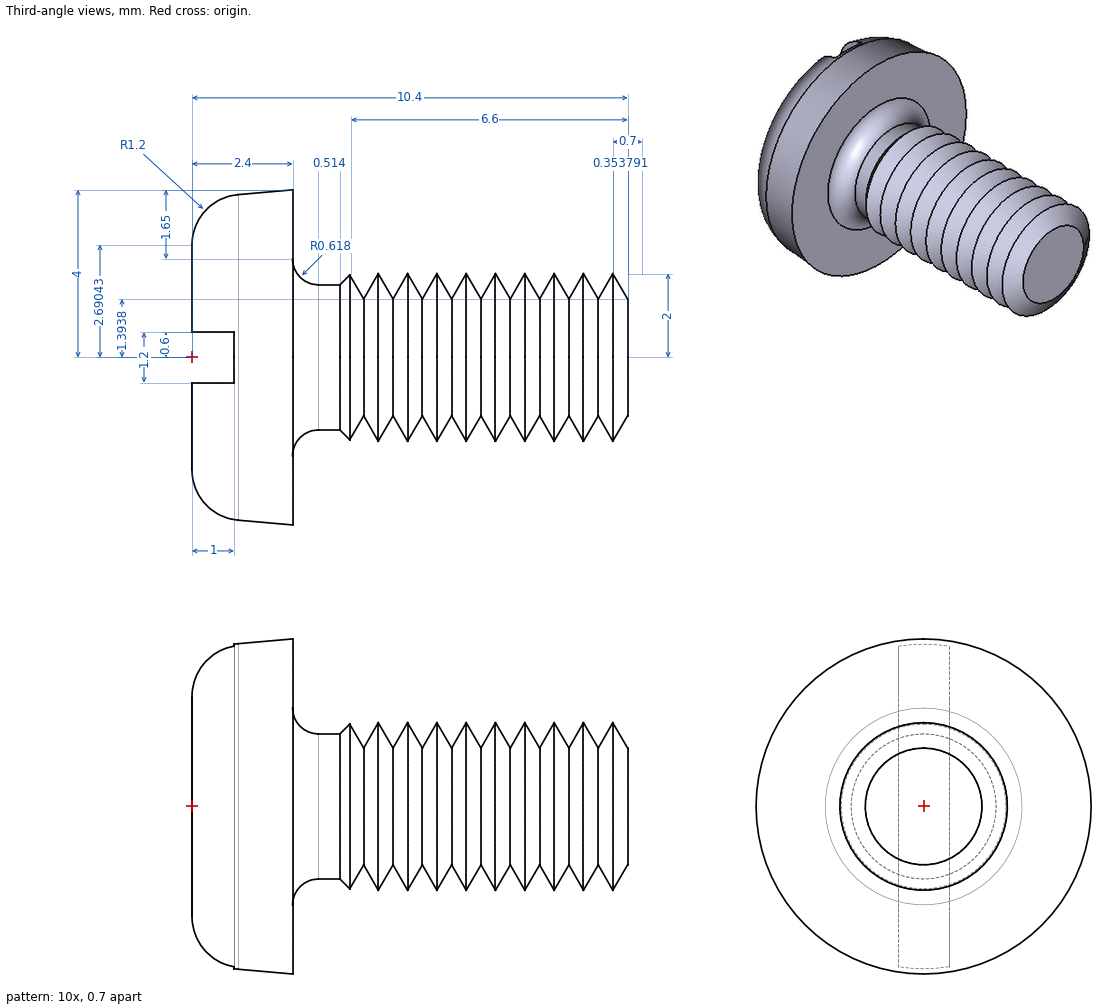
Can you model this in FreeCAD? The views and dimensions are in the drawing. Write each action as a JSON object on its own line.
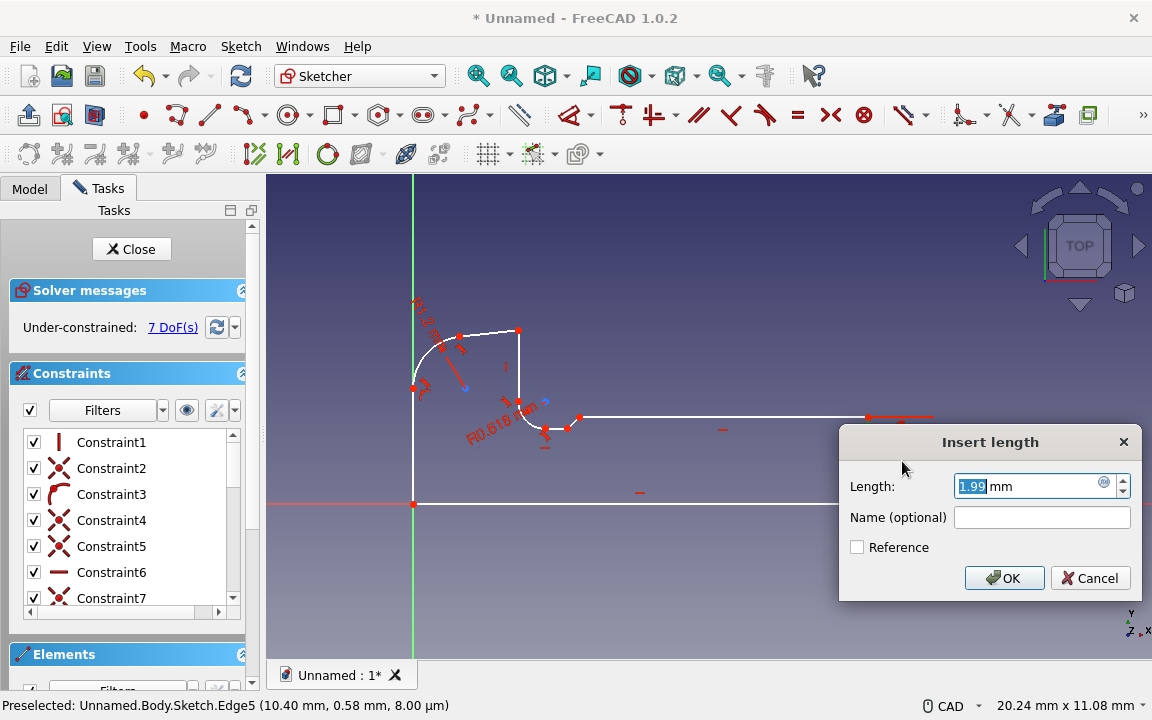
{"action": "type", "text": "2"}
{"action": "key", "text": "Return"}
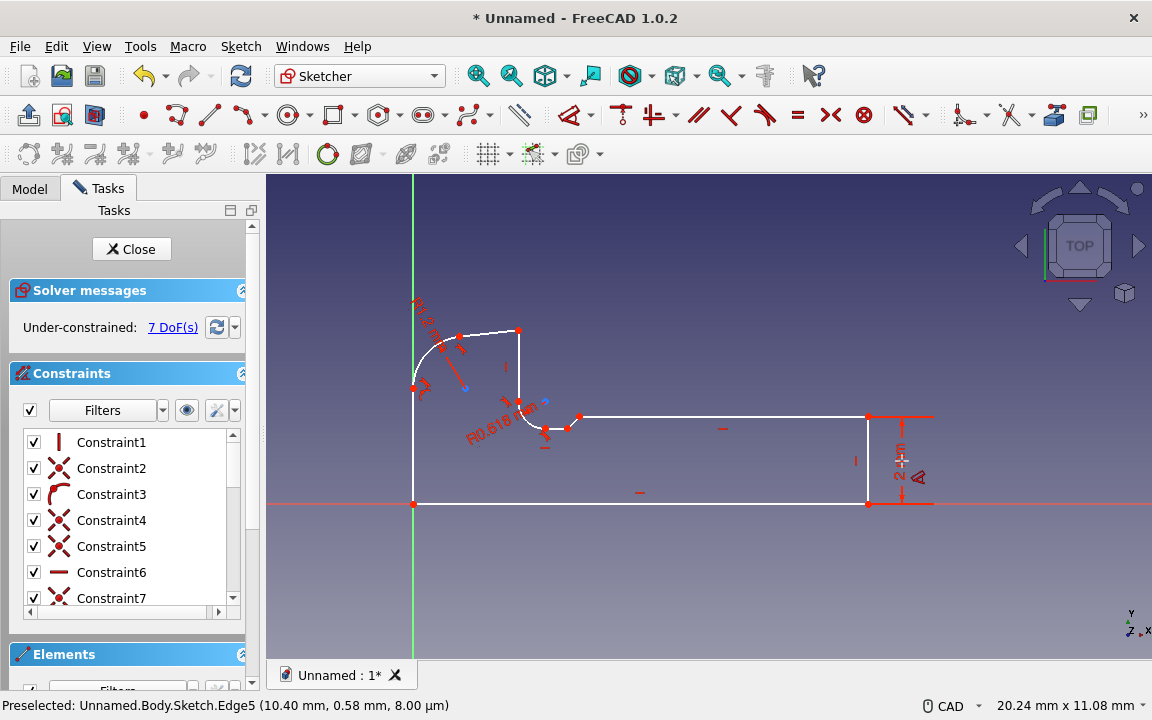
{"action": "left_click", "coordinate": [519, 330]}
{"action": "left_click", "coordinate": [379, 417]}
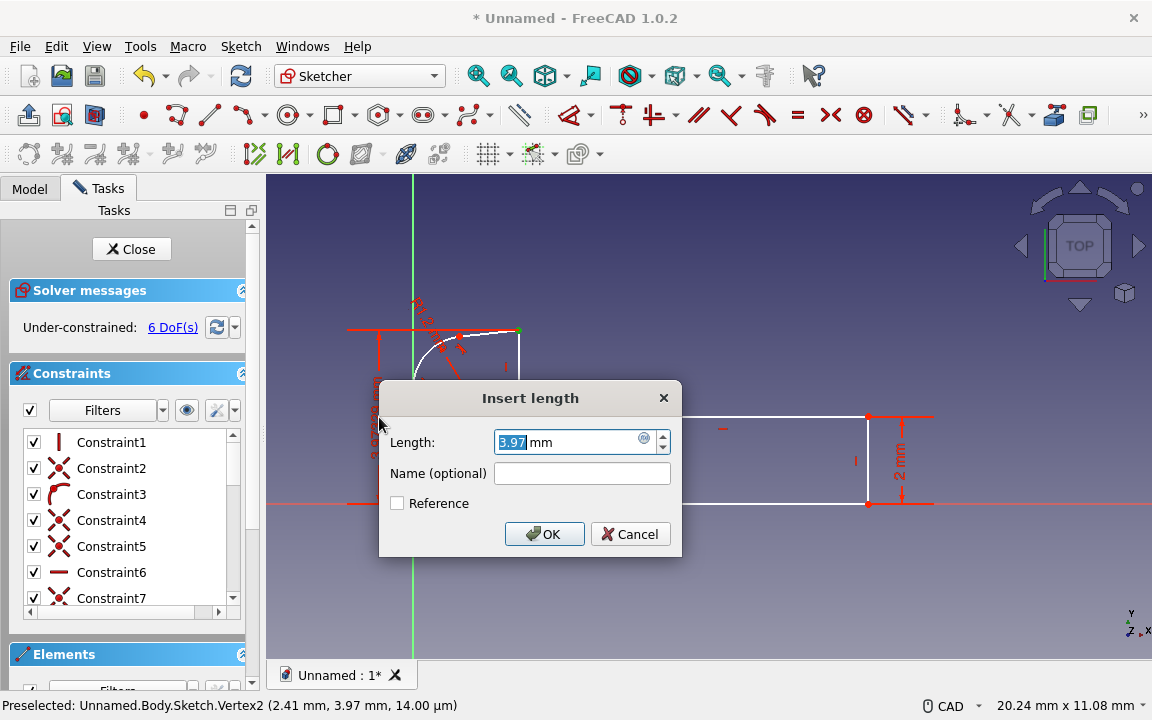
{"action": "type", "text": "4"}
{"action": "key", "text": "Return"}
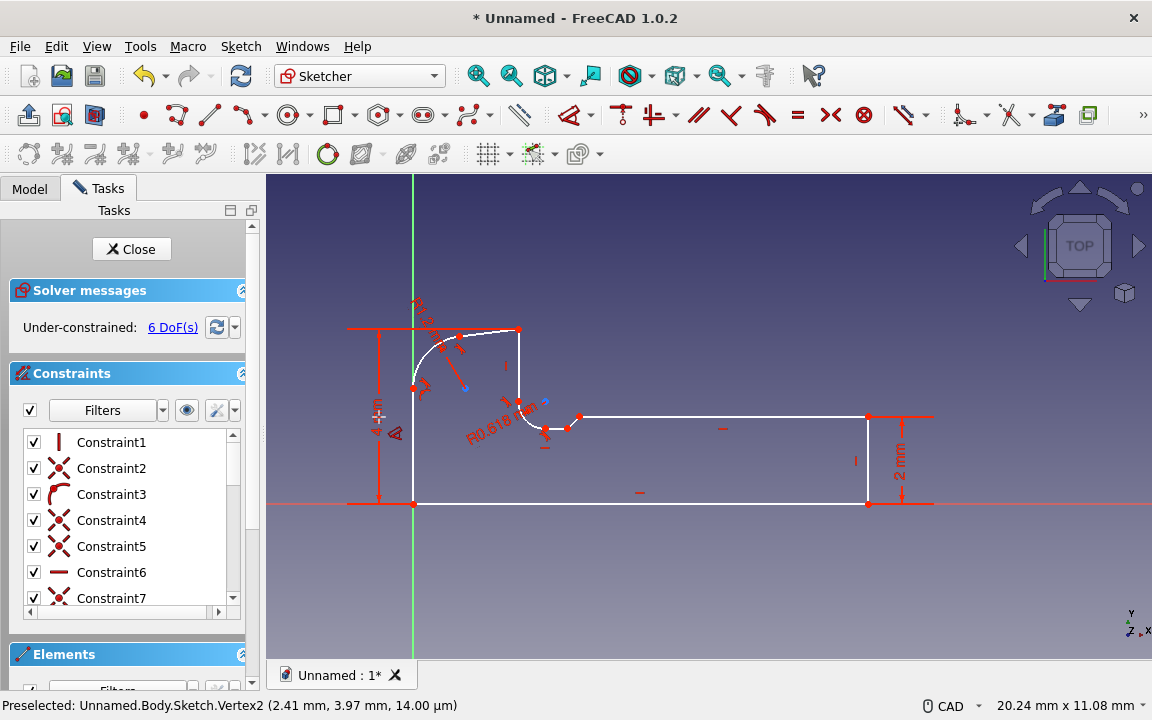
{"action": "left_click", "coordinate": [782, 417]}
{"action": "left_click", "coordinate": [724, 451]}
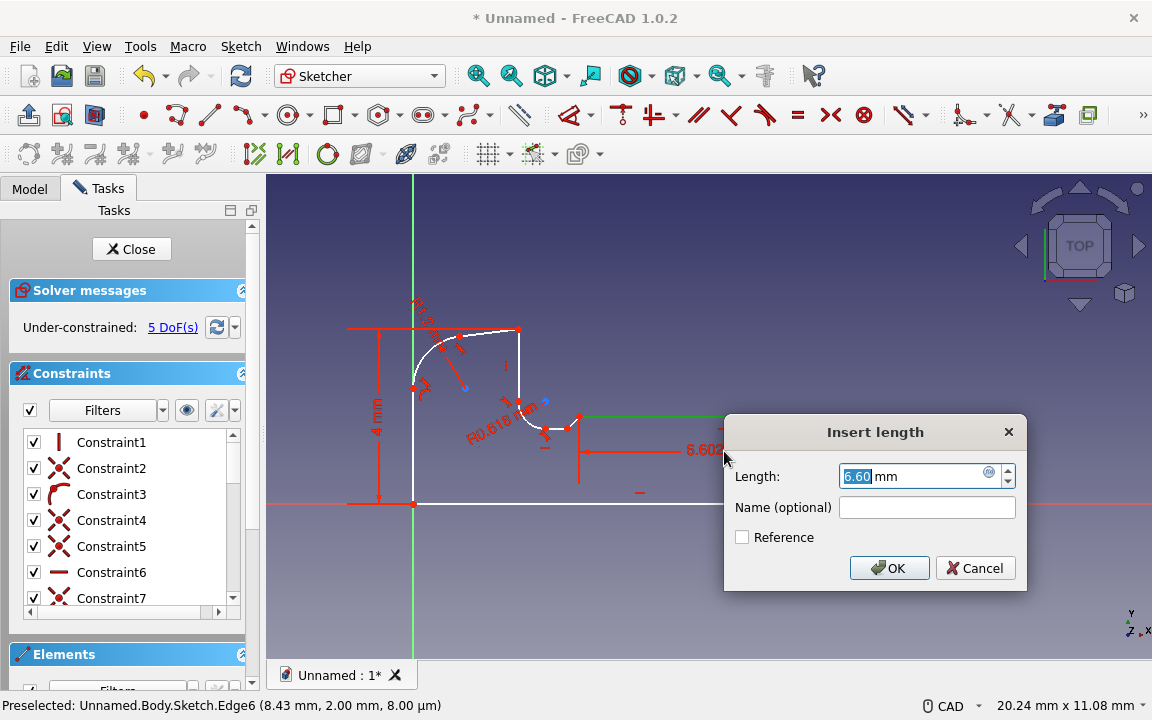
{"action": "type", "text": "6.6"}
{"action": "key", "text": "Return"}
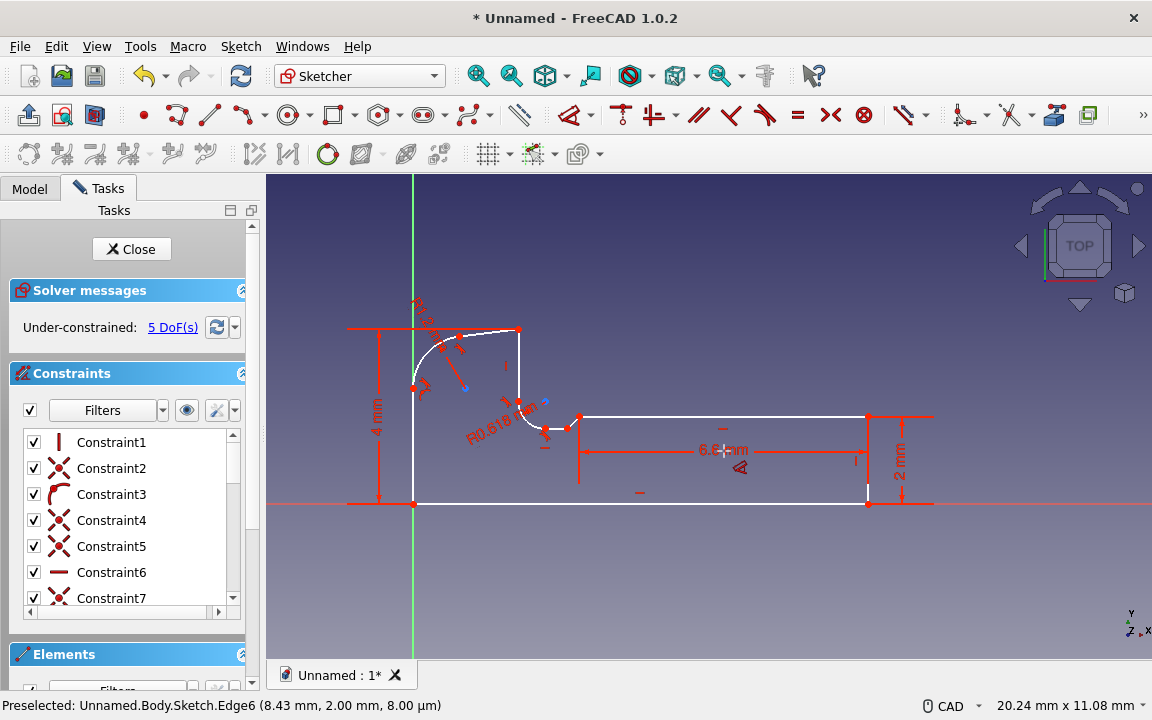
{"action": "left_click", "coordinate": [519, 380]}
{"action": "left_click", "coordinate": [485, 366]}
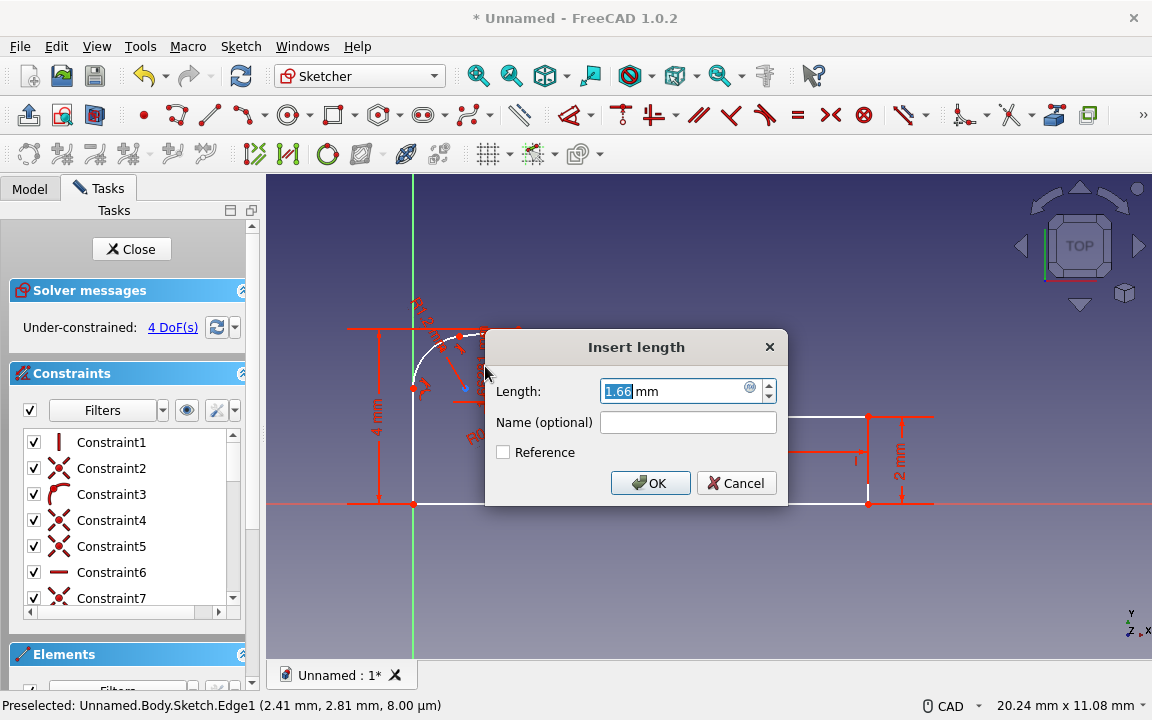
{"action": "type", "text": "1.65"}
{"action": "key", "text": "Return"}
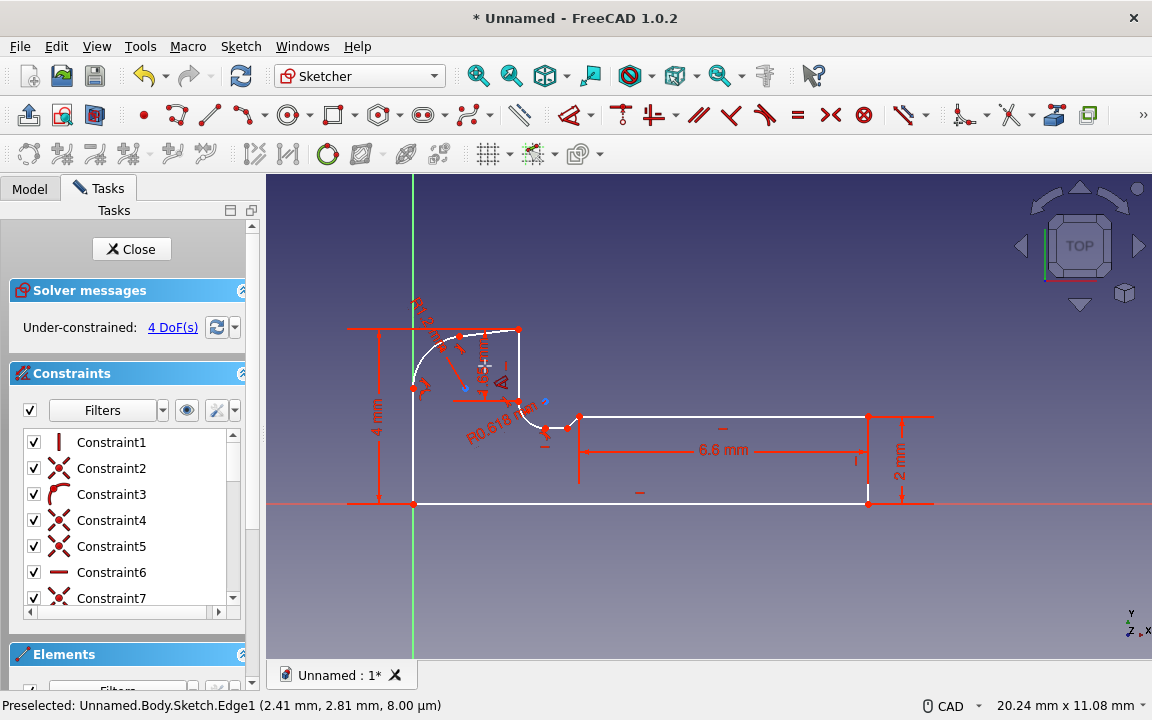
{"action": "left_click", "coordinate": [550, 504]}
{"action": "left_click", "coordinate": [641, 538]}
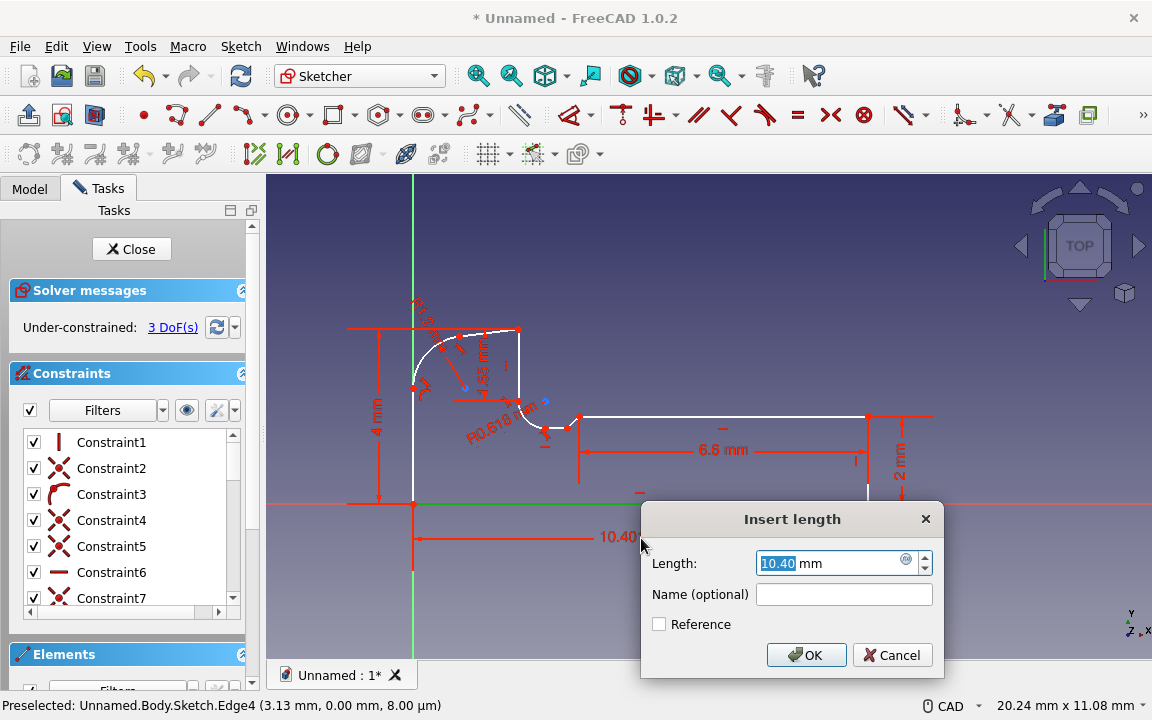
{"action": "type", "text": "10.4"}
{"action": "key", "text": "Return"}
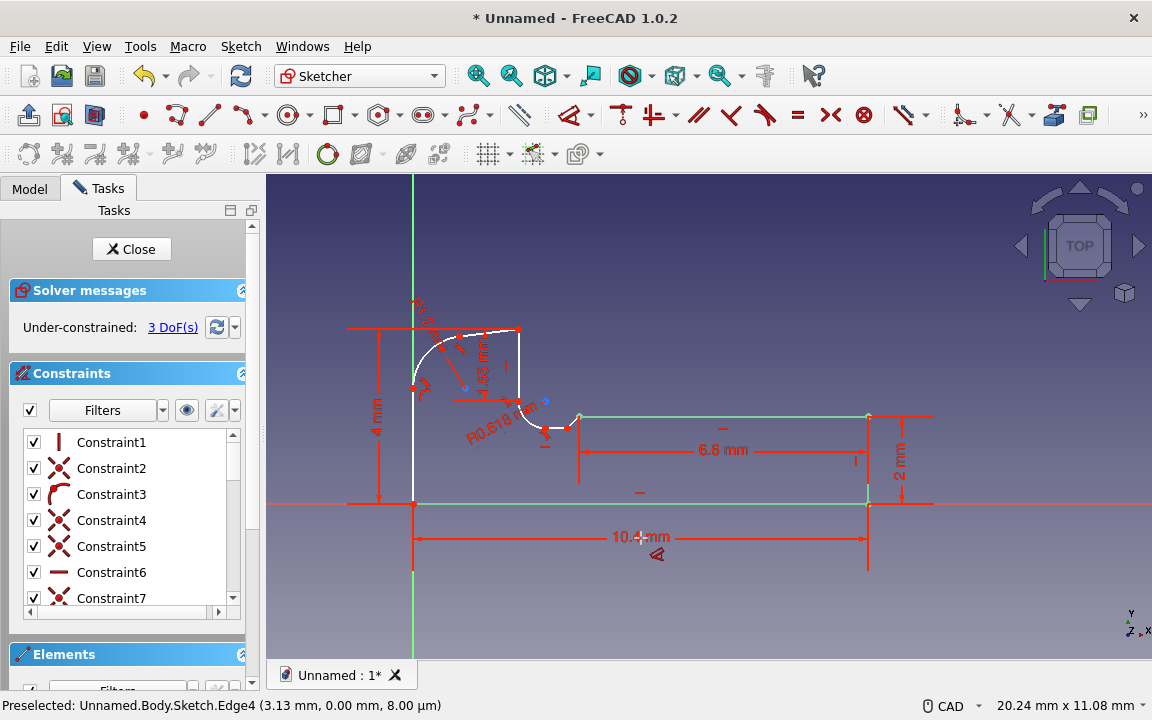
{"action": "left_click", "coordinate": [519, 401]}
{"action": "left_click", "coordinate": [466, 538]}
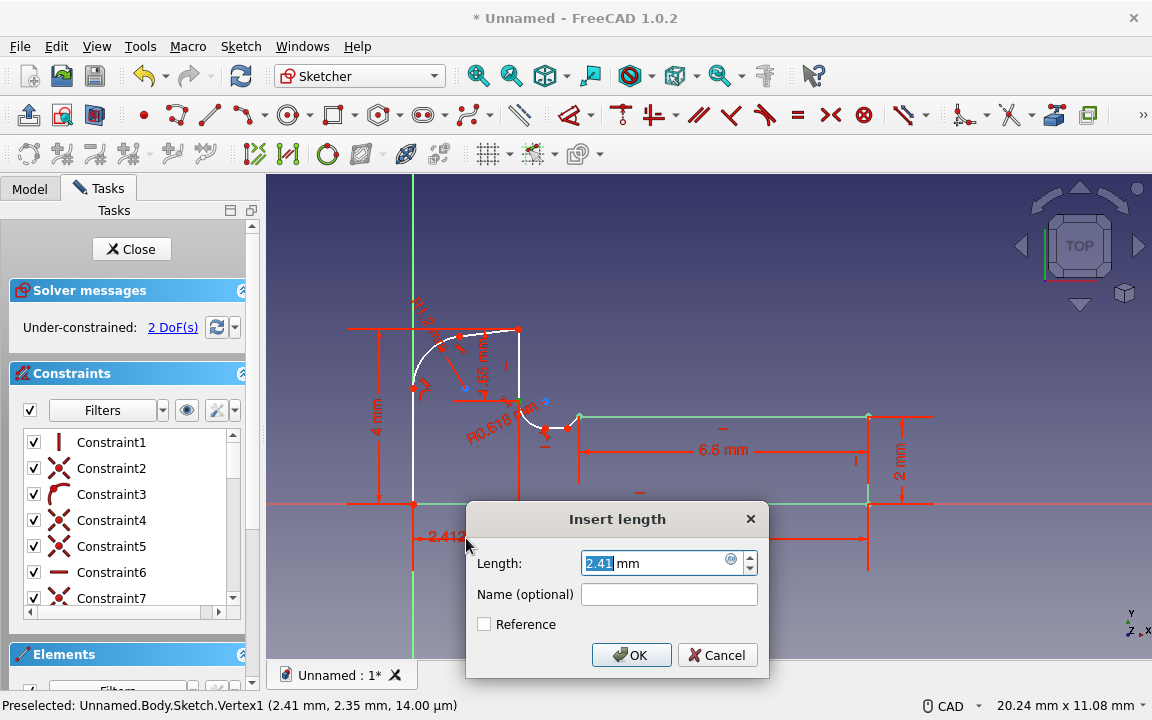
{"action": "type", "text": "2.4"}
{"action": "key", "text": "Return"}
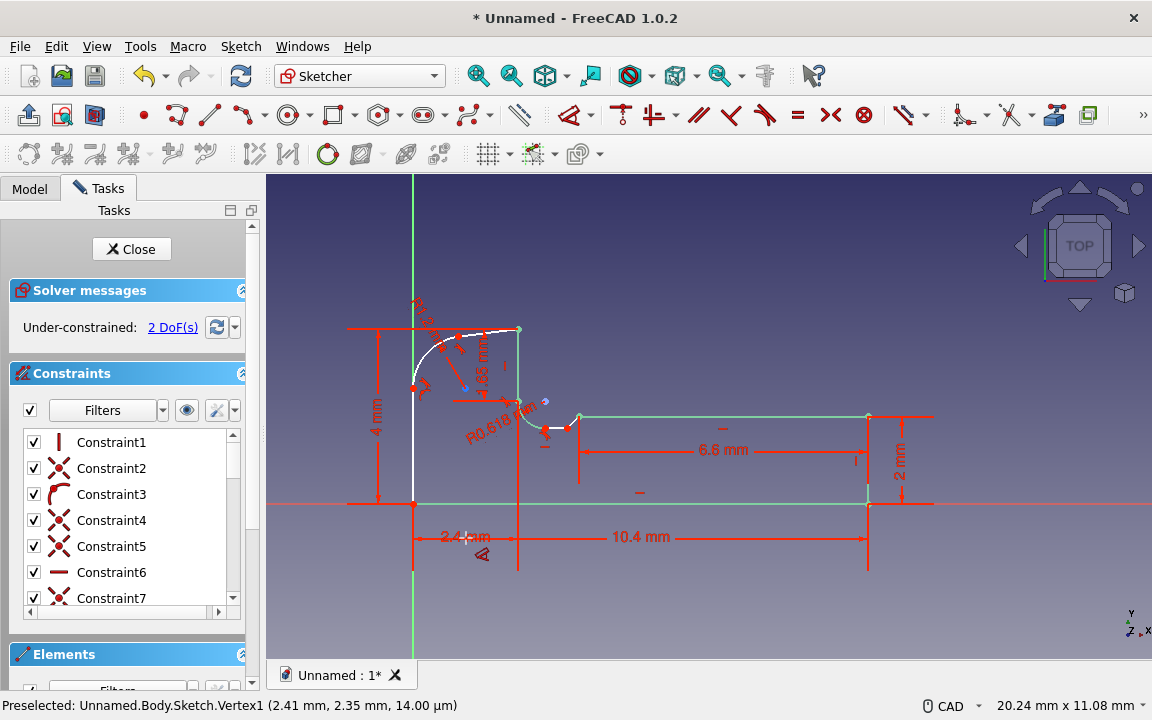
{"action": "scroll", "coordinate": [556, 428], "scroll_direction": "up", "scroll_amount": 3}